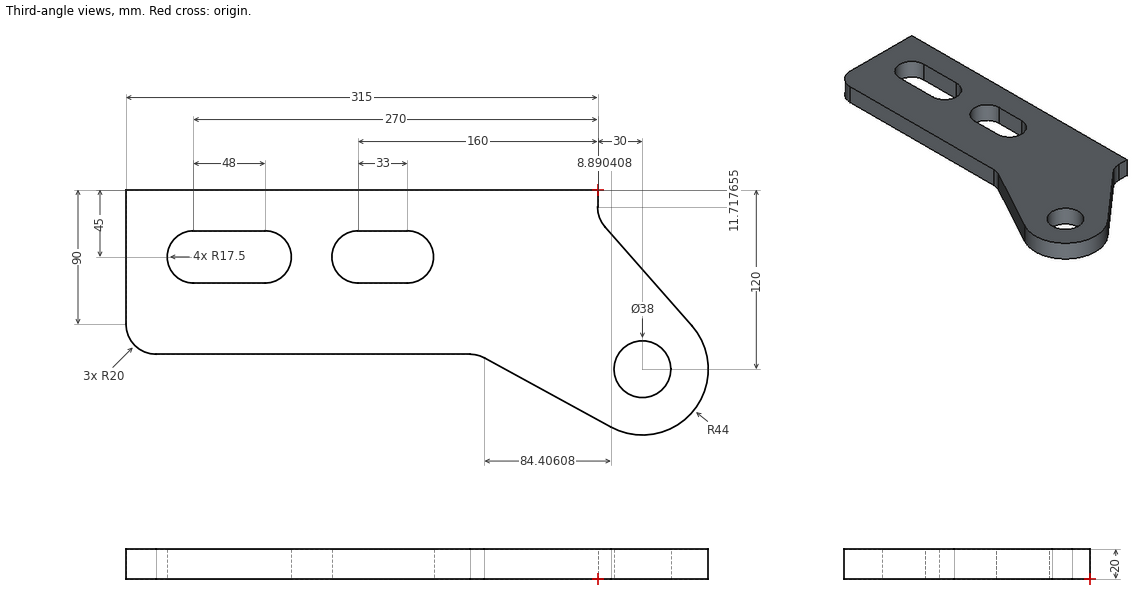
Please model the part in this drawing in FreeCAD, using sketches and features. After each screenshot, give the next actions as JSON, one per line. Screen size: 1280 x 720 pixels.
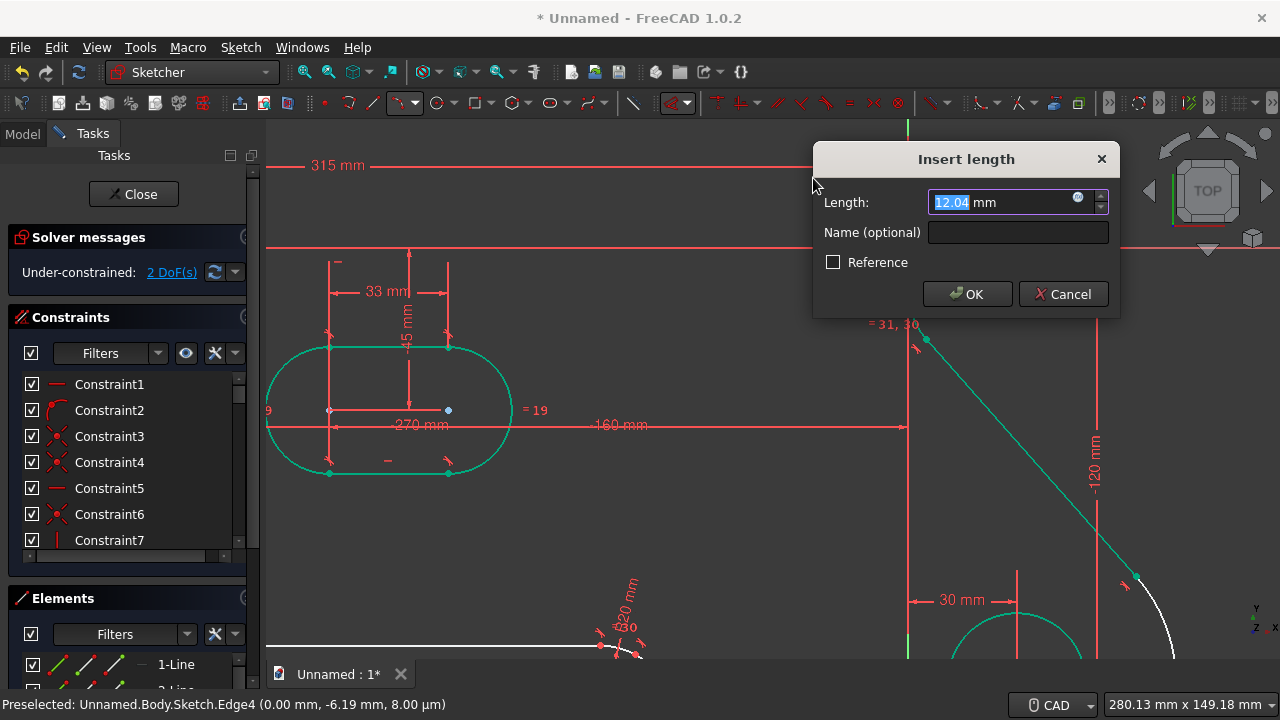
{"action": "type", "text": "11.717655"}
{"action": "key", "text": "Return"}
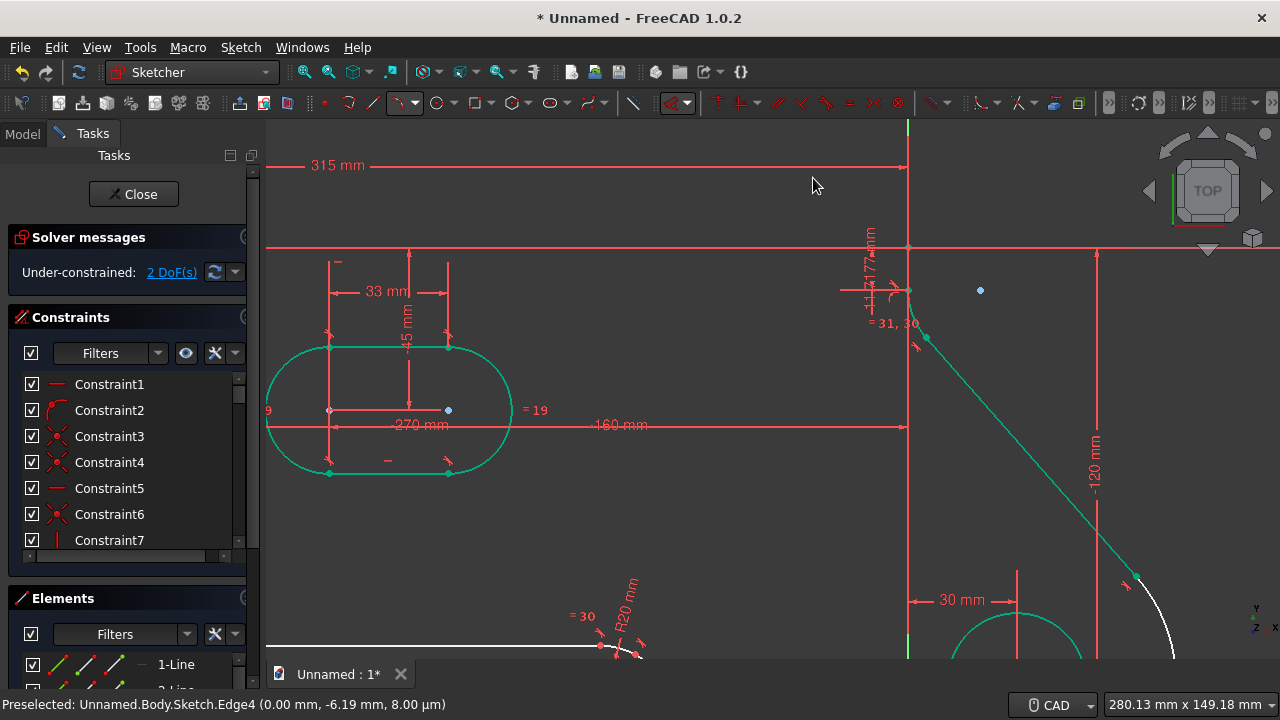
{"action": "scroll", "coordinate": [908, 270], "scroll_direction": "down", "scroll_amount": 4}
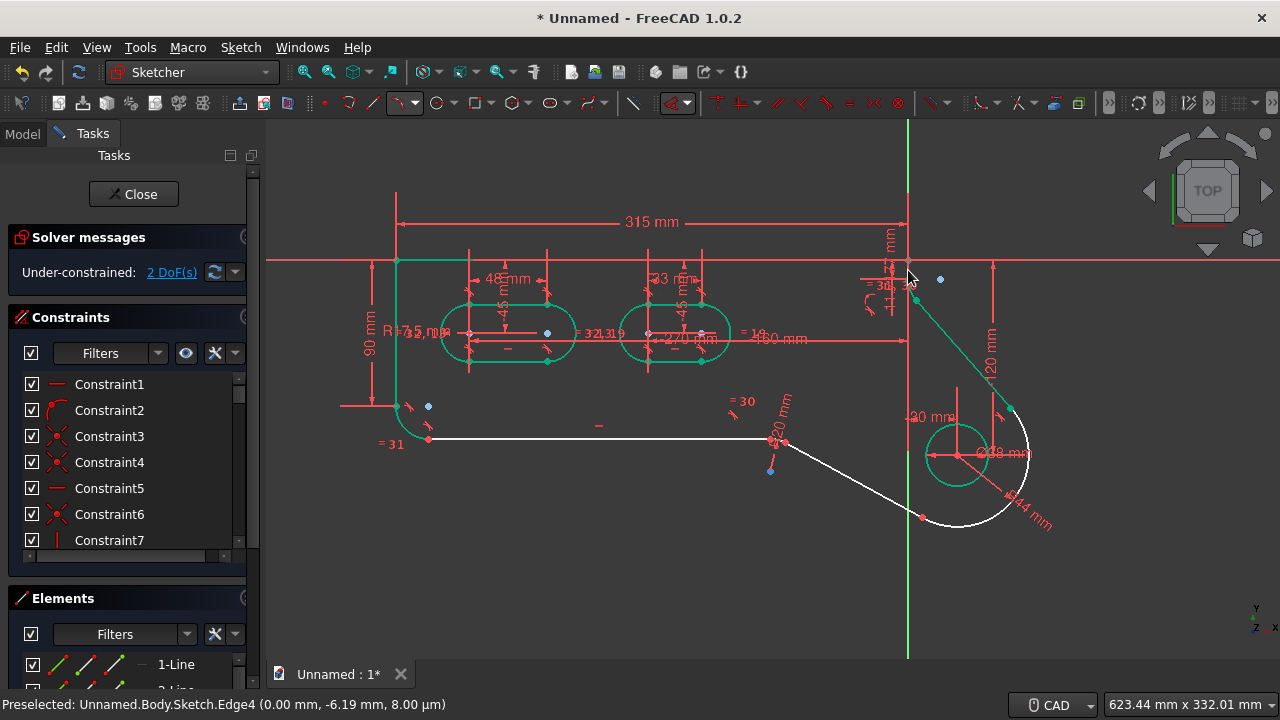
{"action": "scroll", "coordinate": [923, 518], "scroll_direction": "up", "scroll_amount": 6}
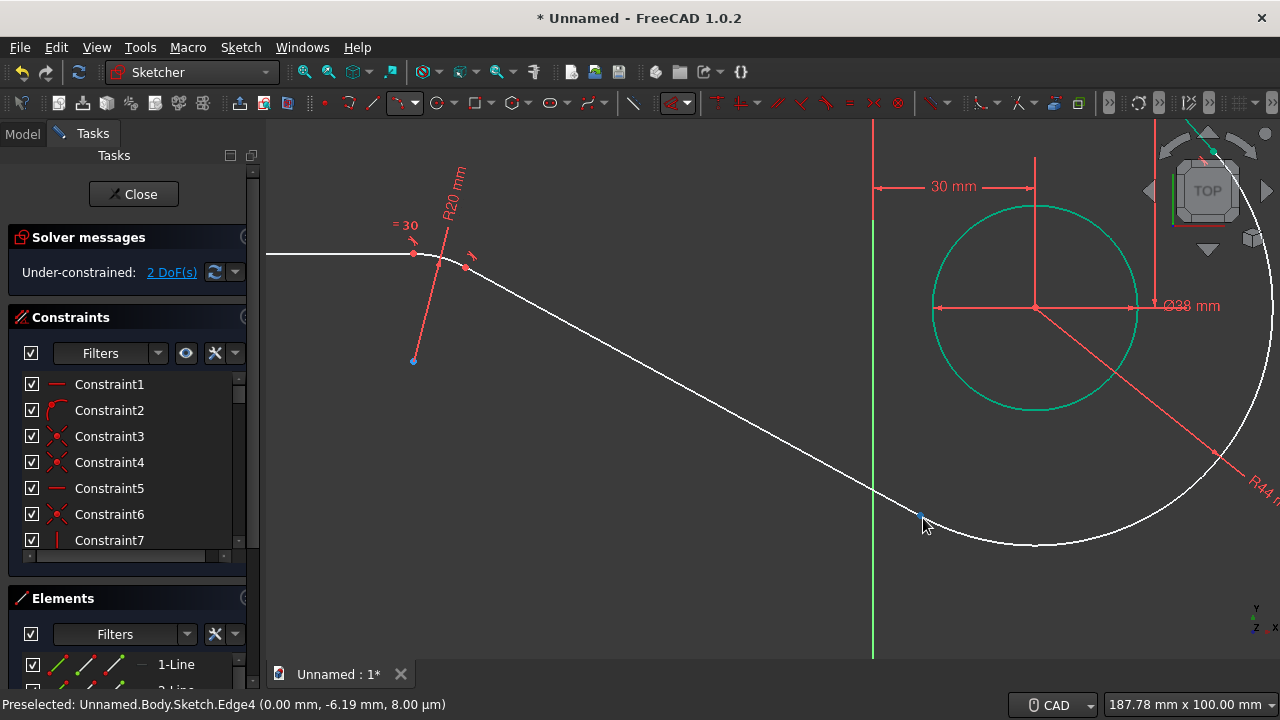
{"action": "left_click", "coordinate": [920, 516]}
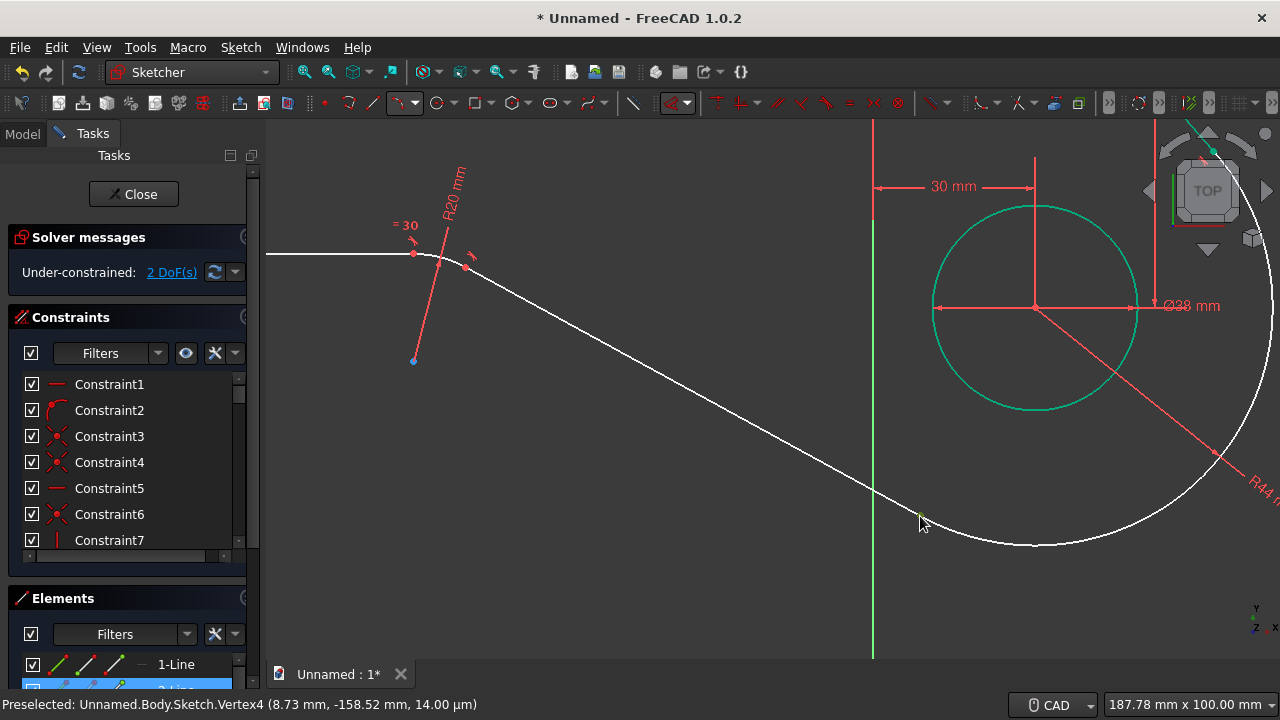
{"action": "left_click", "coordinate": [690, 104]}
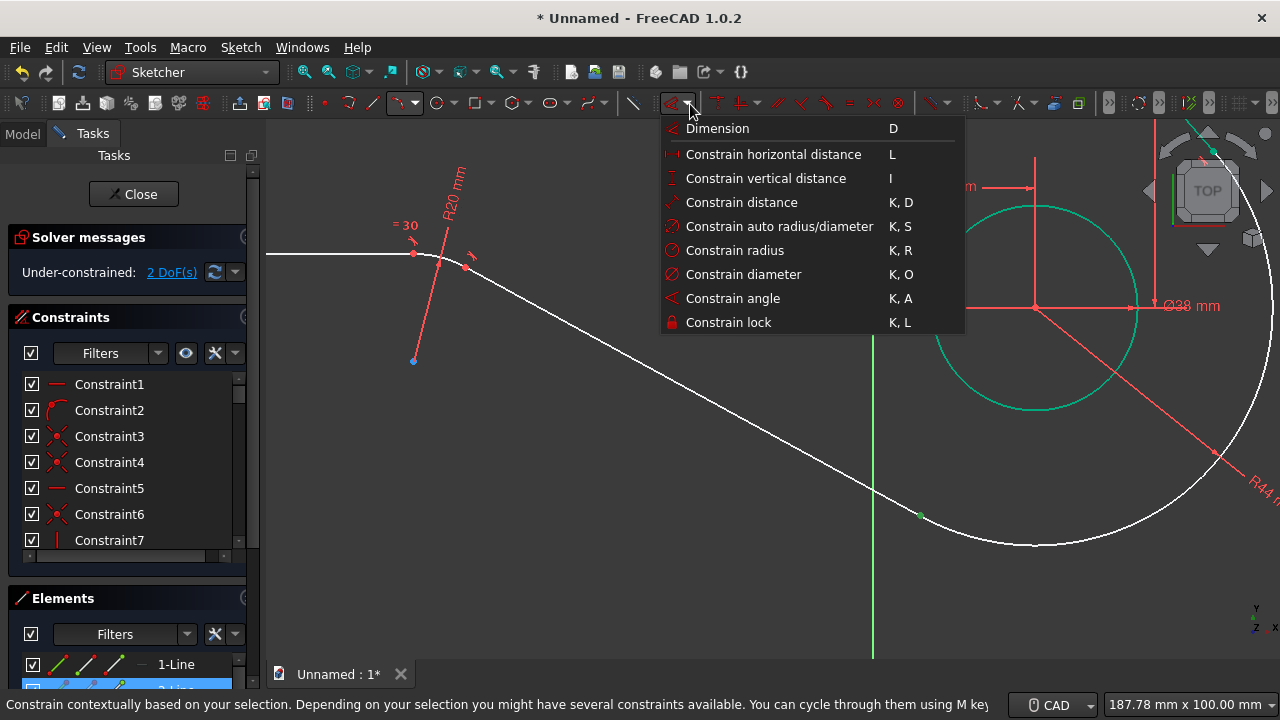
{"action": "left_click", "coordinate": [813, 154]}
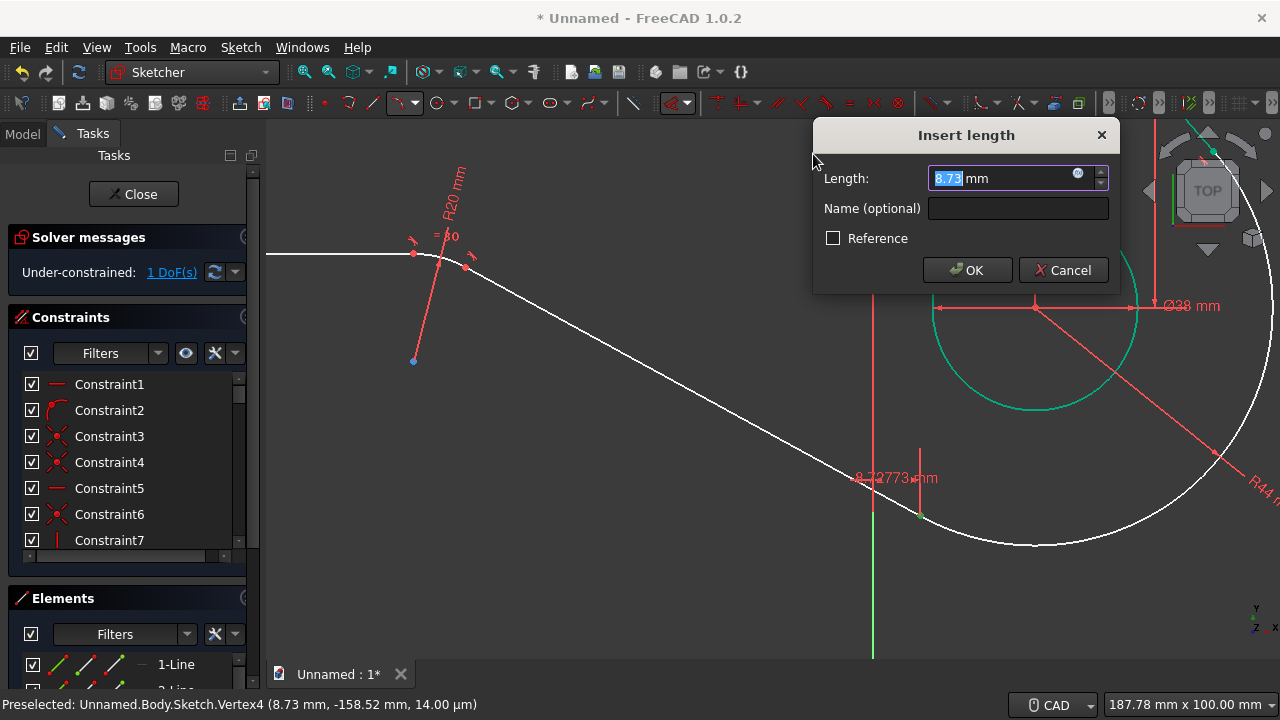
{"action": "type", "text": "8.890408"}
{"action": "key", "text": "Return"}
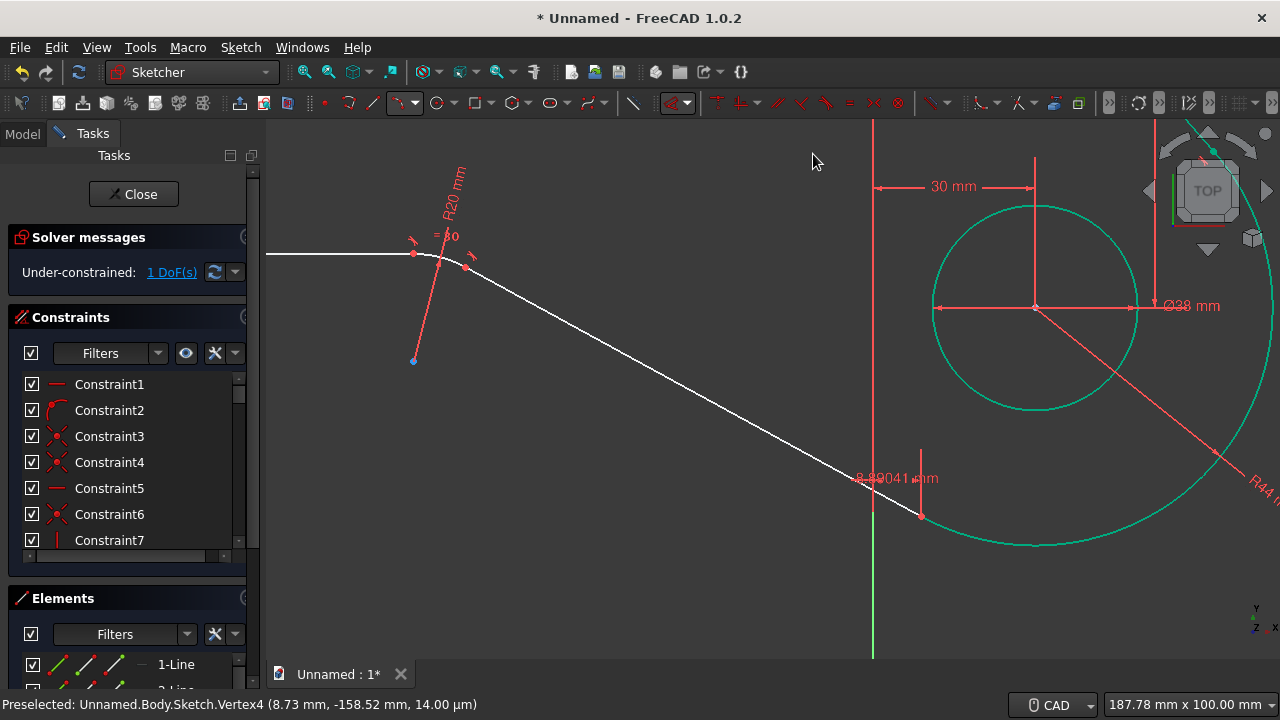
{"action": "left_click", "coordinate": [602, 342]}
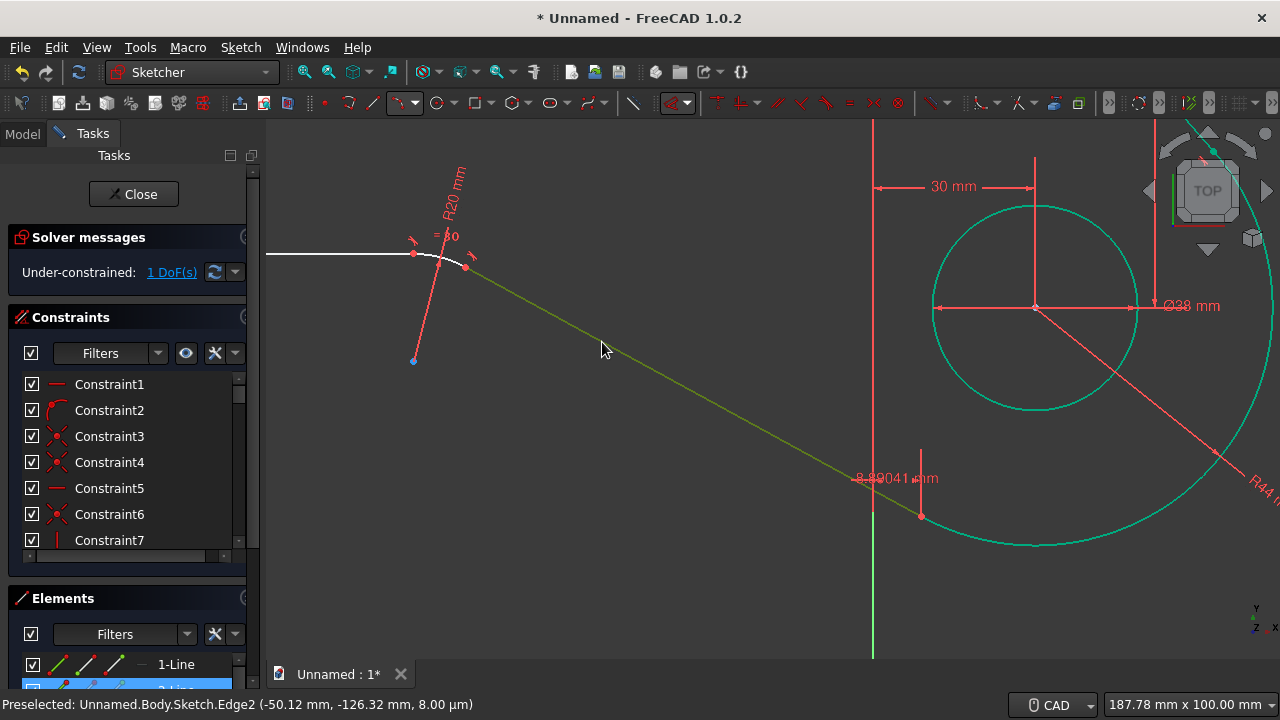
{"action": "key", "text": "l"}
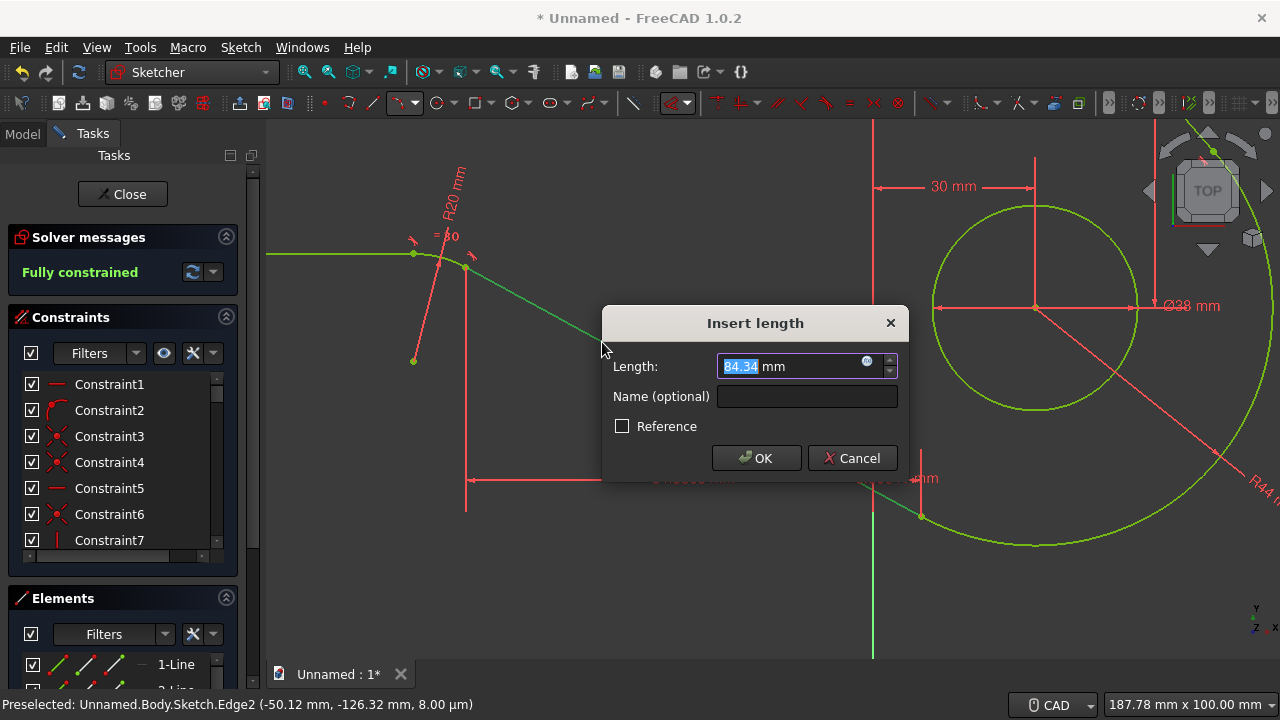
{"action": "type", "text": "84.40608"}
{"action": "key", "text": "Return"}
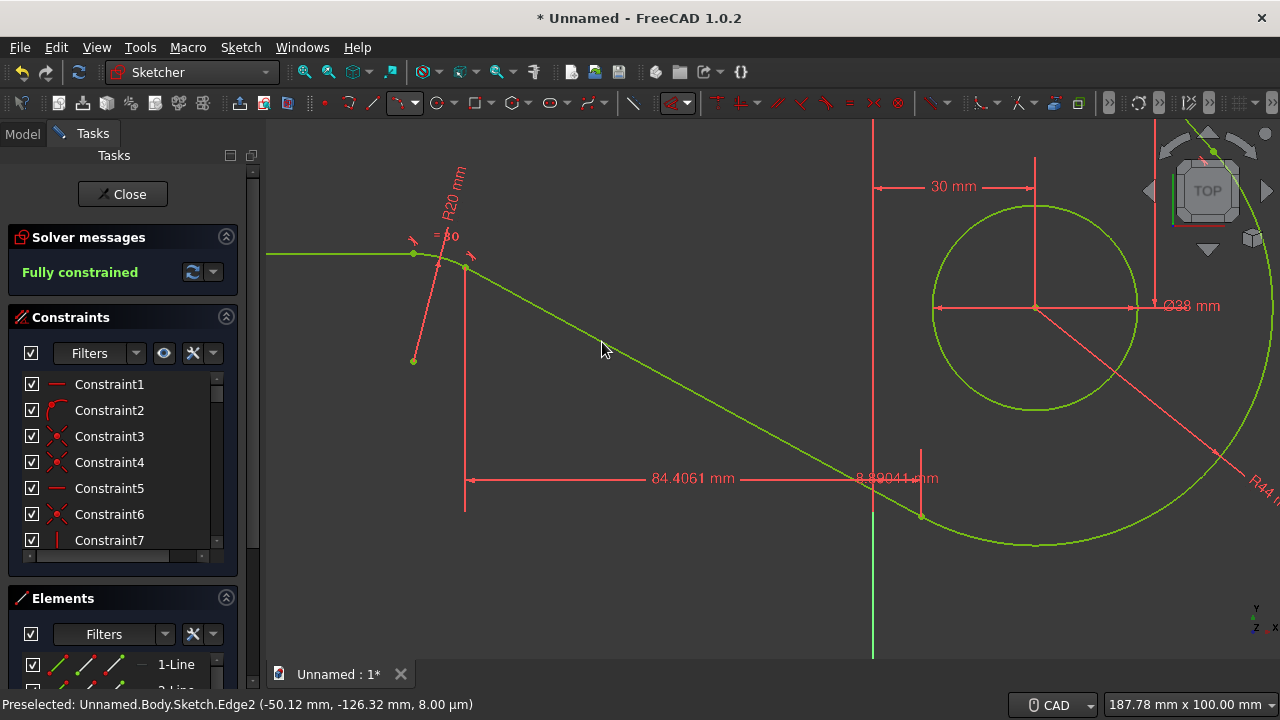
{"action": "left_click", "coordinate": [123, 194]}